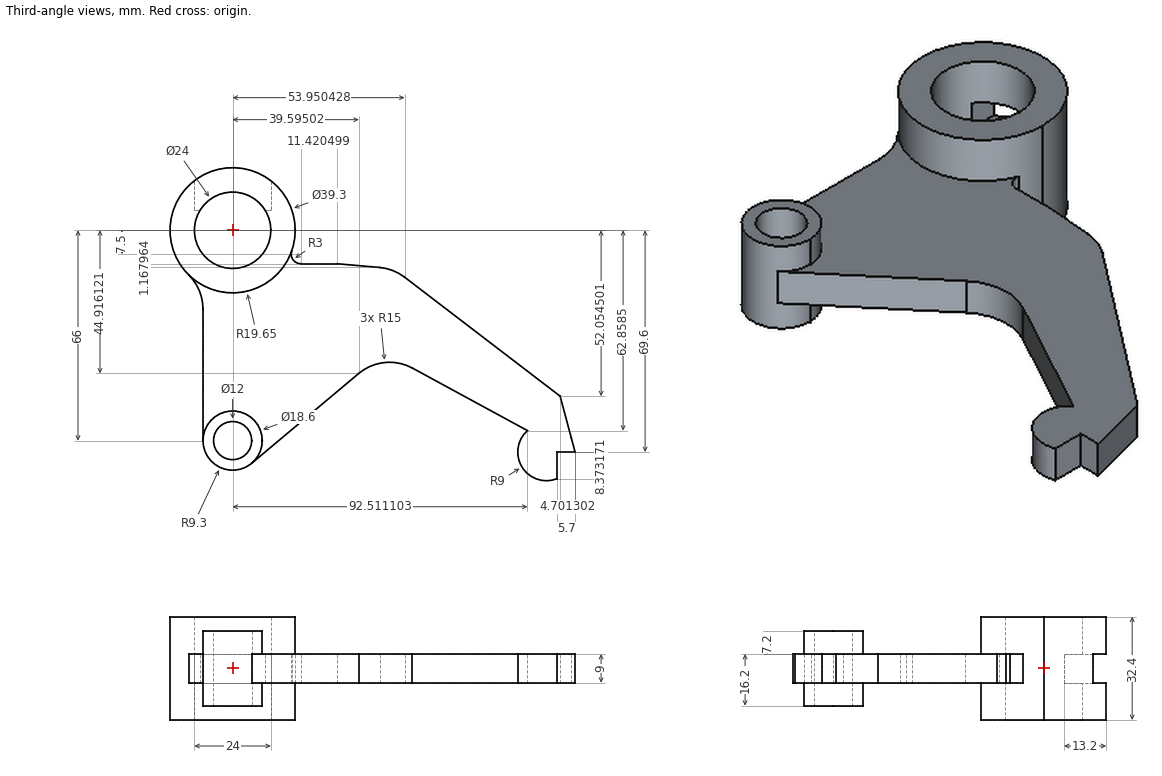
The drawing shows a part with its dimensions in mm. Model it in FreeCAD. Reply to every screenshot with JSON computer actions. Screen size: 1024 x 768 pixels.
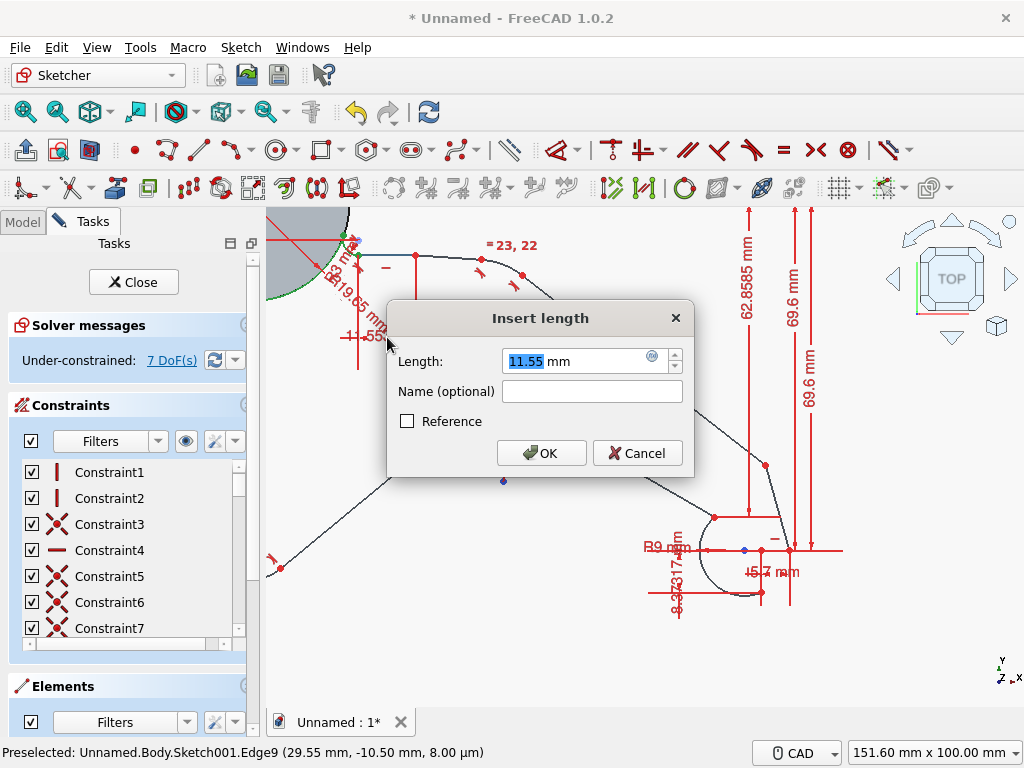
{"action": "type", "text": "11.420499"}
{"action": "key", "text": "Return"}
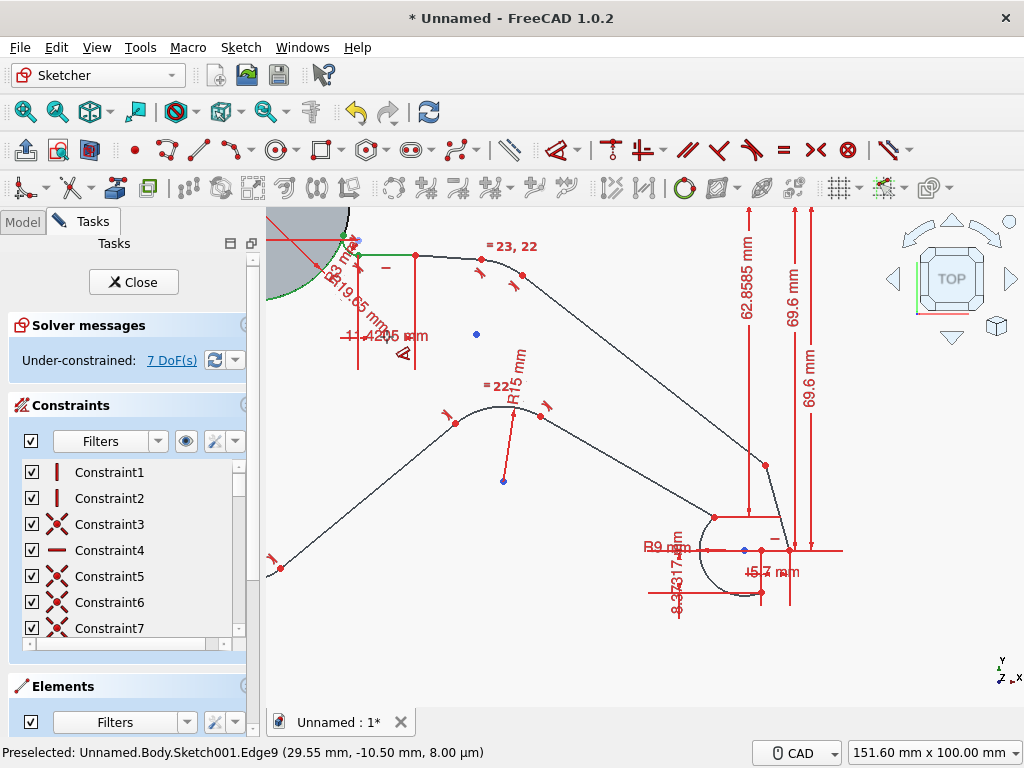
{"action": "left_click", "coordinate": [456, 424]}
{"action": "left_click", "coordinate": [375, 458]}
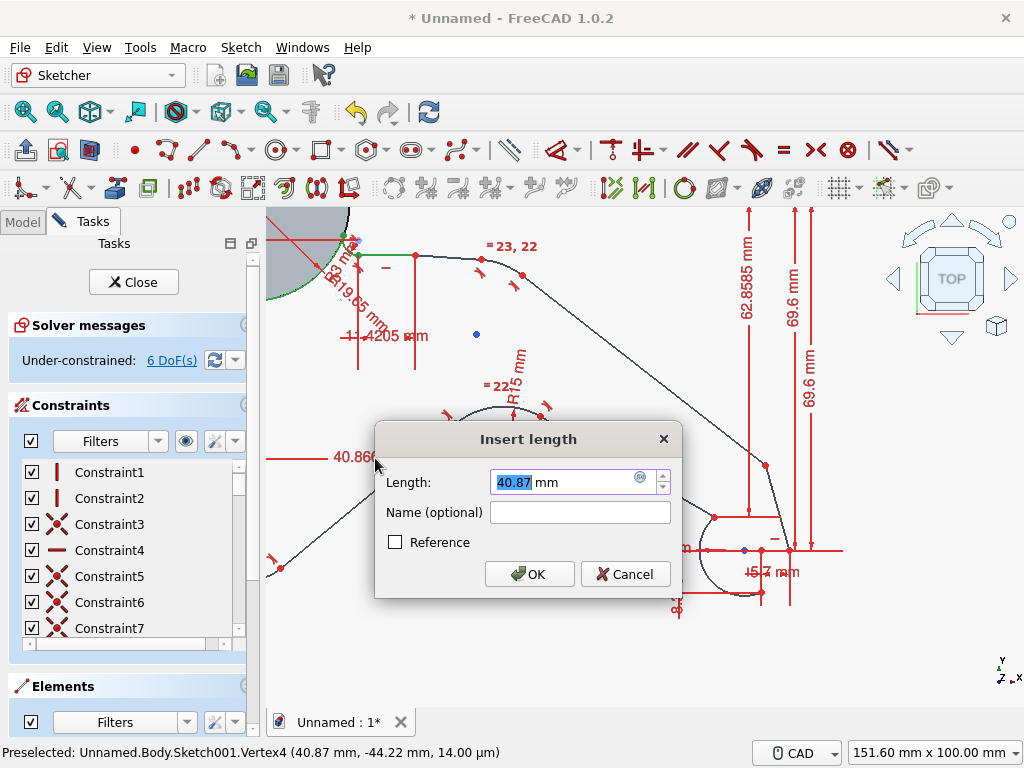
{"action": "type", "text": "39.59502"}
{"action": "key", "text": "Return"}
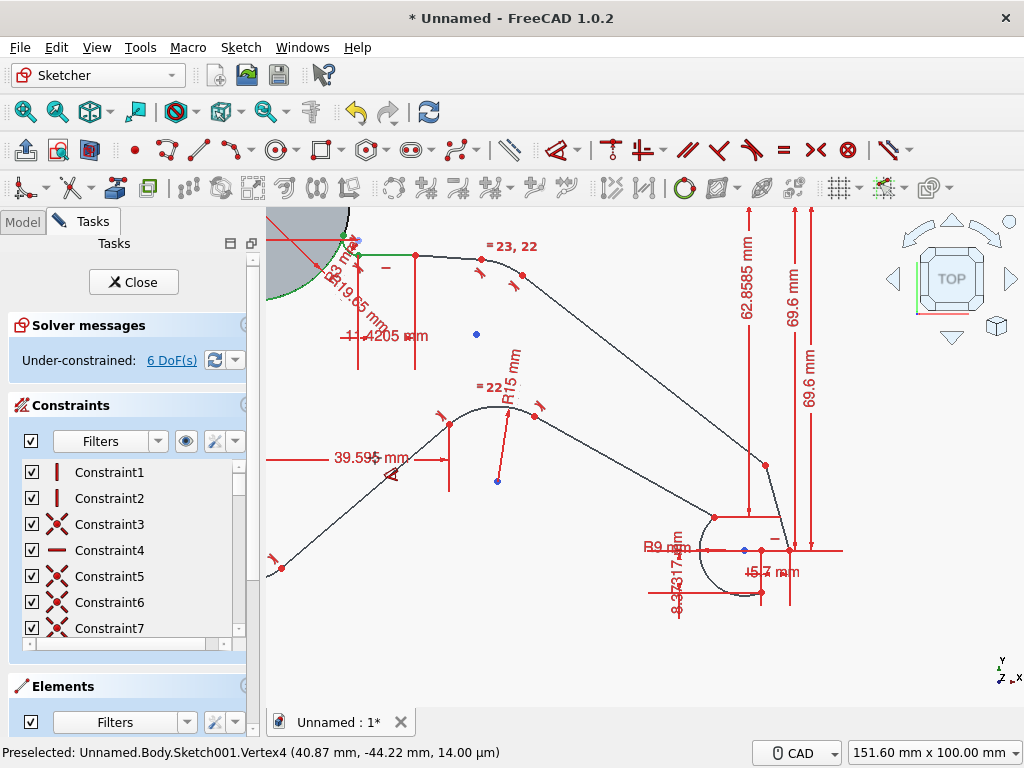
{"action": "scroll", "coordinate": [782, 525], "scroll_direction": "up", "scroll_amount": 3}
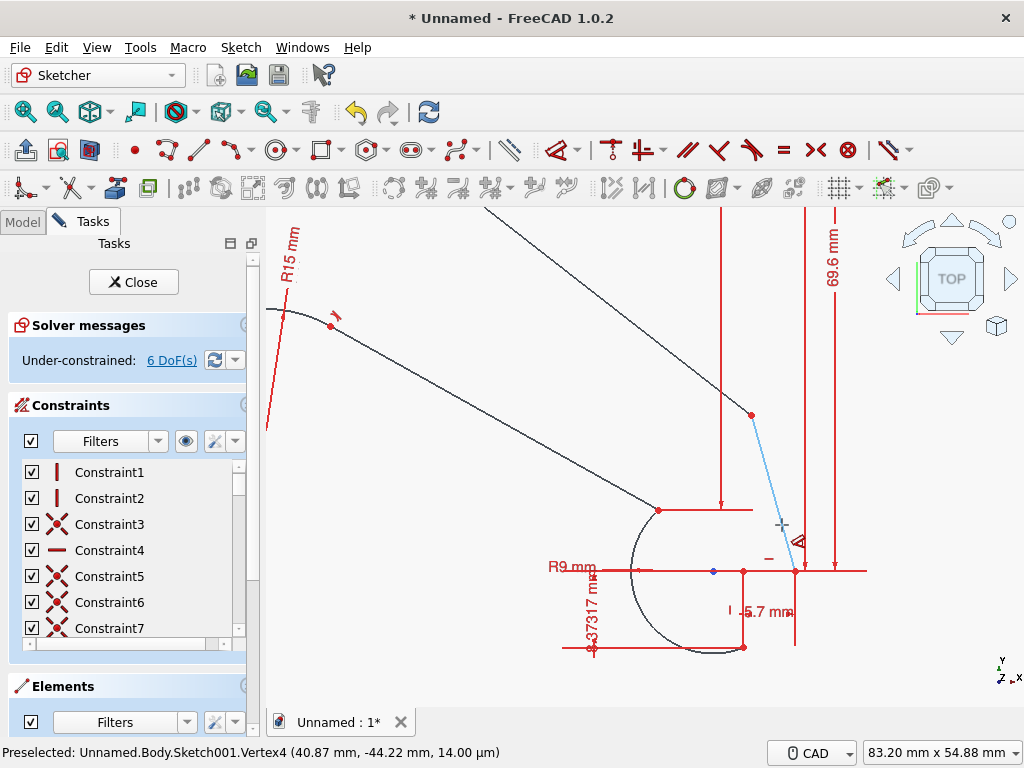
{"action": "left_click", "coordinate": [782, 525]}
{"action": "left_click", "coordinate": [773, 382]}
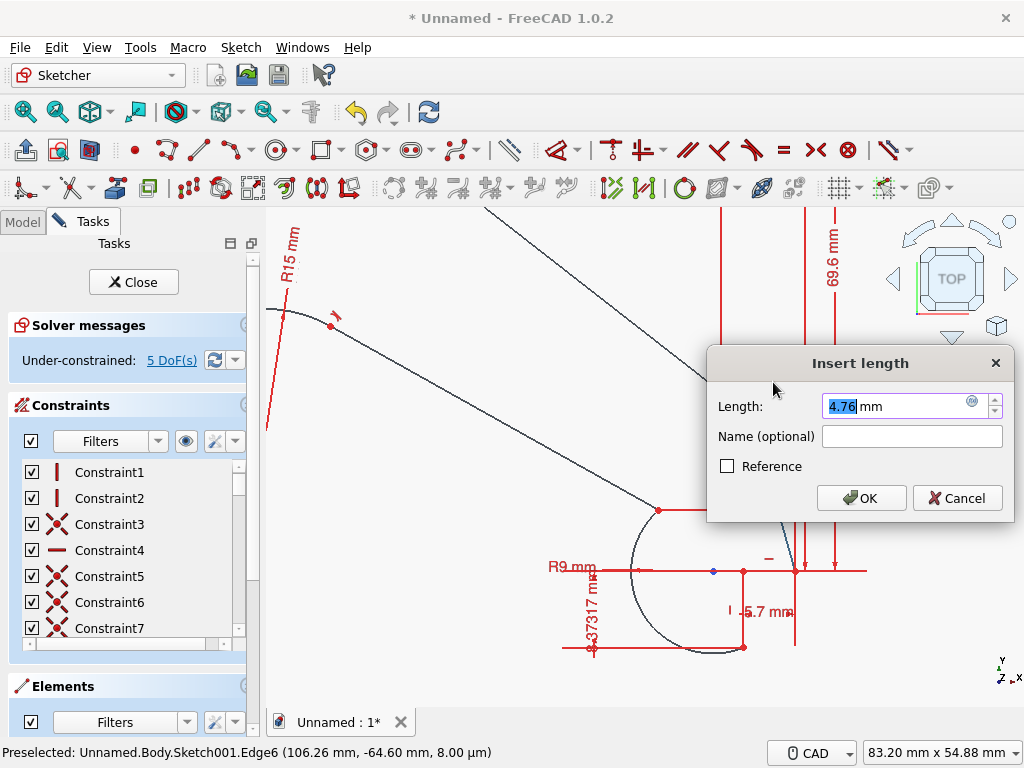
{"action": "type", "text": "4.701302"}
{"action": "key", "text": "Return"}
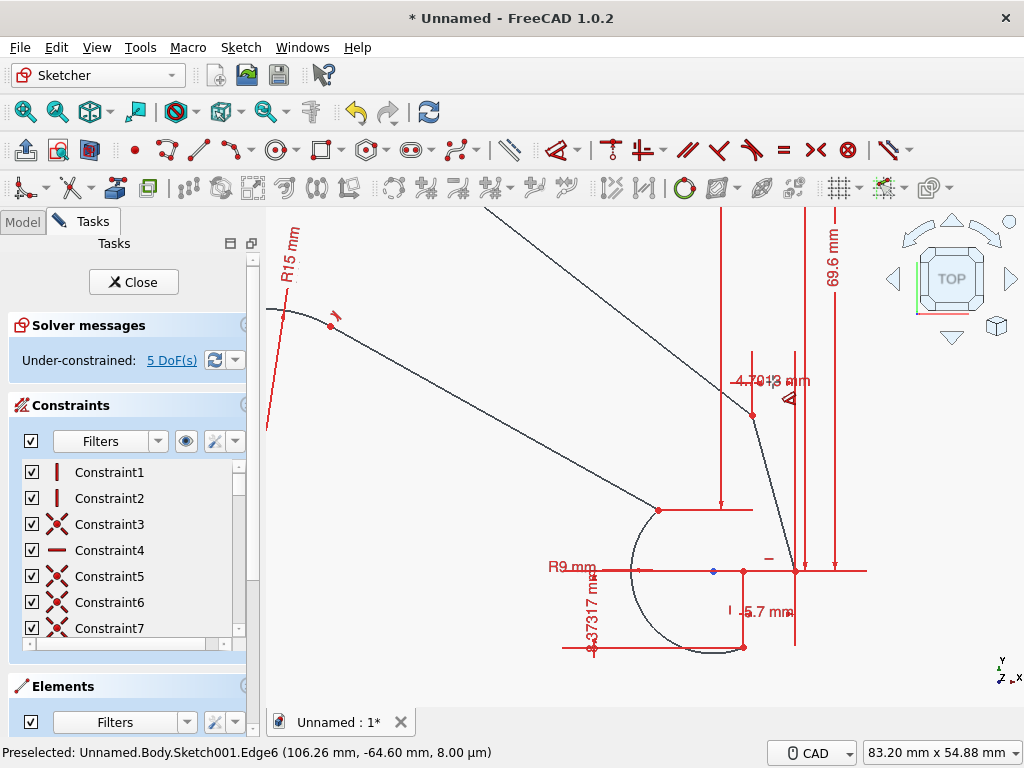
{"action": "scroll", "coordinate": [772, 553], "scroll_direction": "down", "scroll_amount": 5}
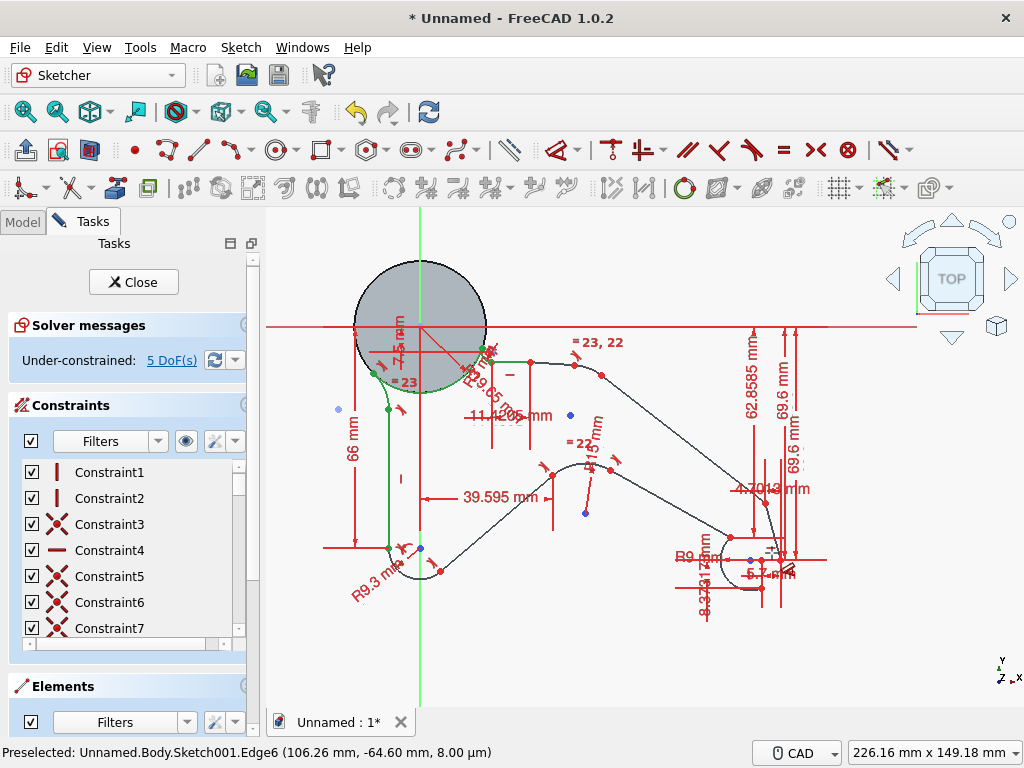
{"action": "scroll", "coordinate": [561, 364], "scroll_direction": "up", "scroll_amount": 12}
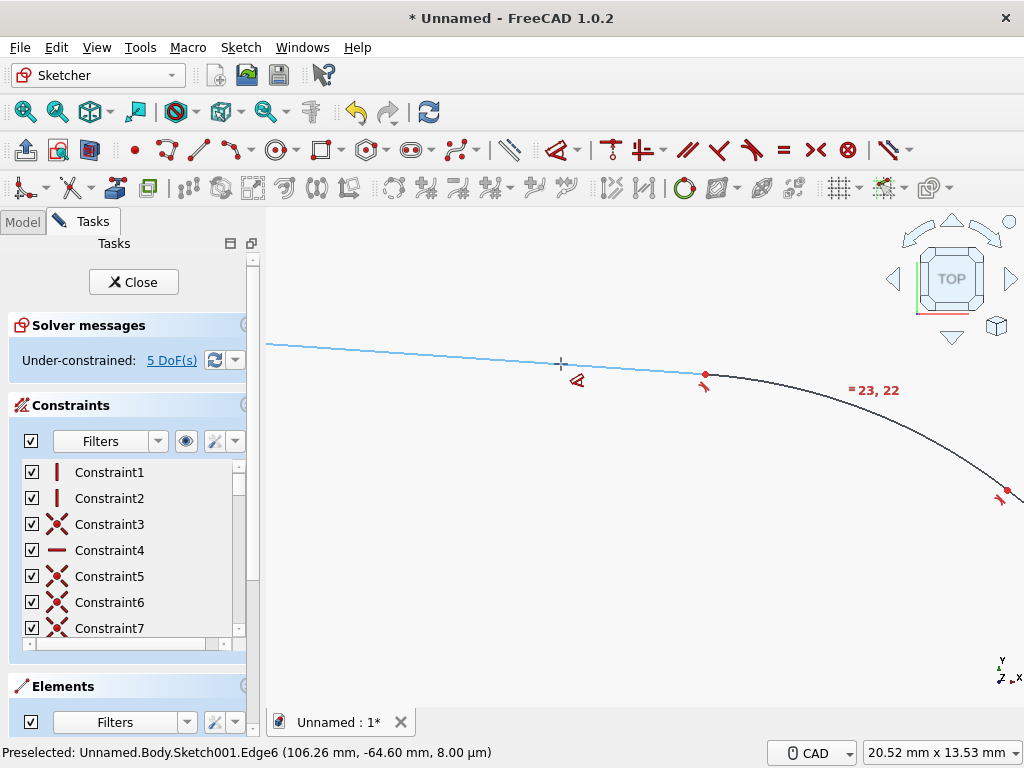
{"action": "left_click", "coordinate": [558, 364]}
{"action": "left_click", "coordinate": [739, 357]}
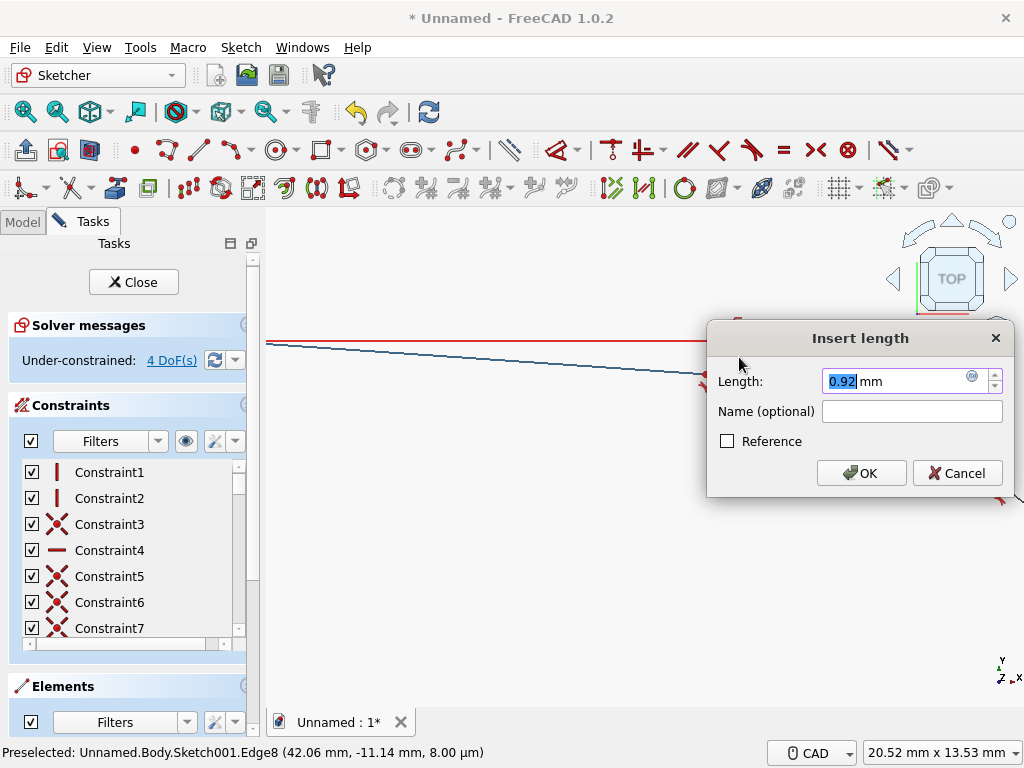
{"action": "type", "text": "1.167964"}
{"action": "key", "text": "Return"}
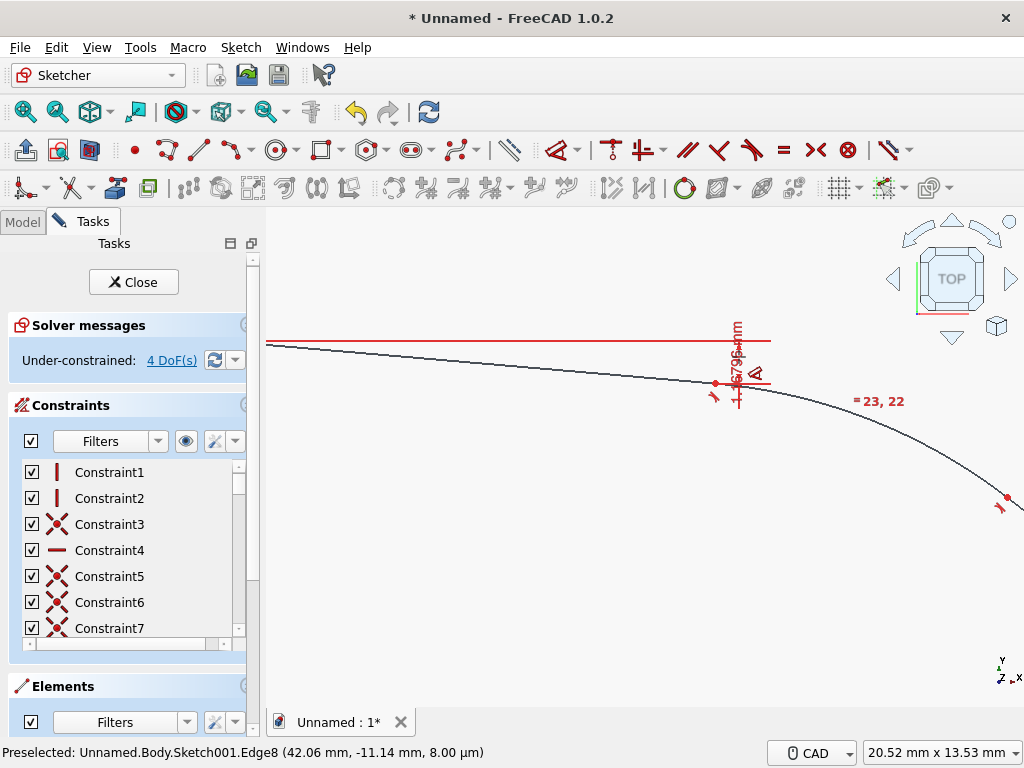
{"action": "scroll", "coordinate": [561, 364], "scroll_direction": "down", "scroll_amount": 12}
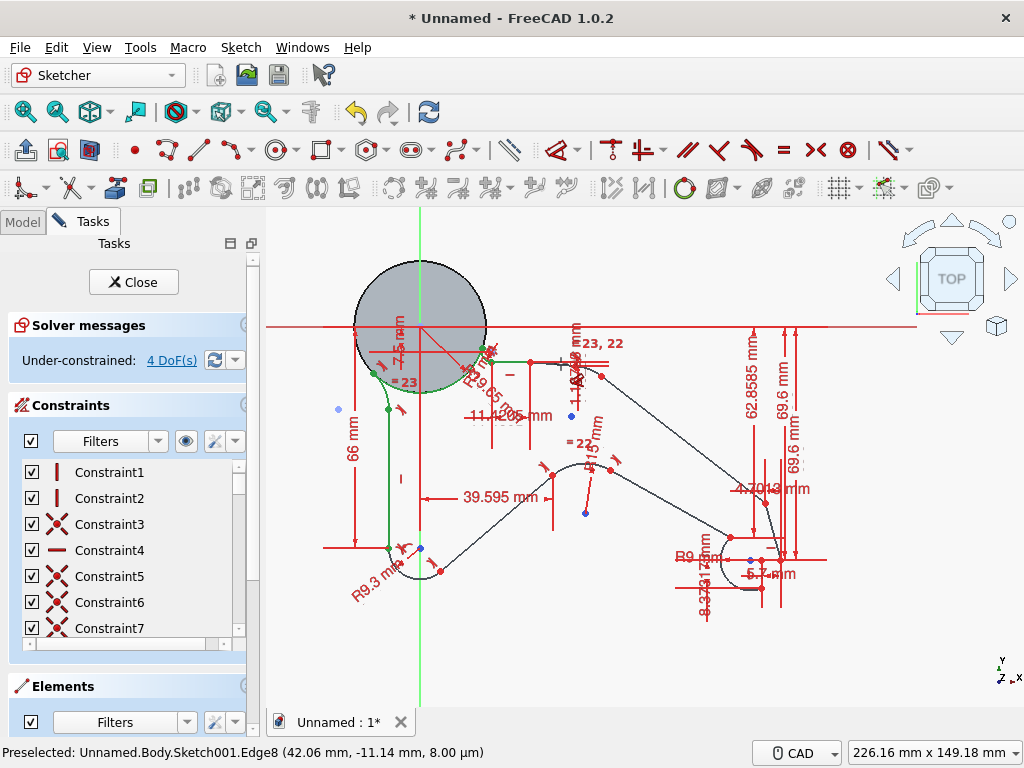
{"action": "left_click", "coordinate": [553, 476]}
{"action": "left_click", "coordinate": [386, 367]}